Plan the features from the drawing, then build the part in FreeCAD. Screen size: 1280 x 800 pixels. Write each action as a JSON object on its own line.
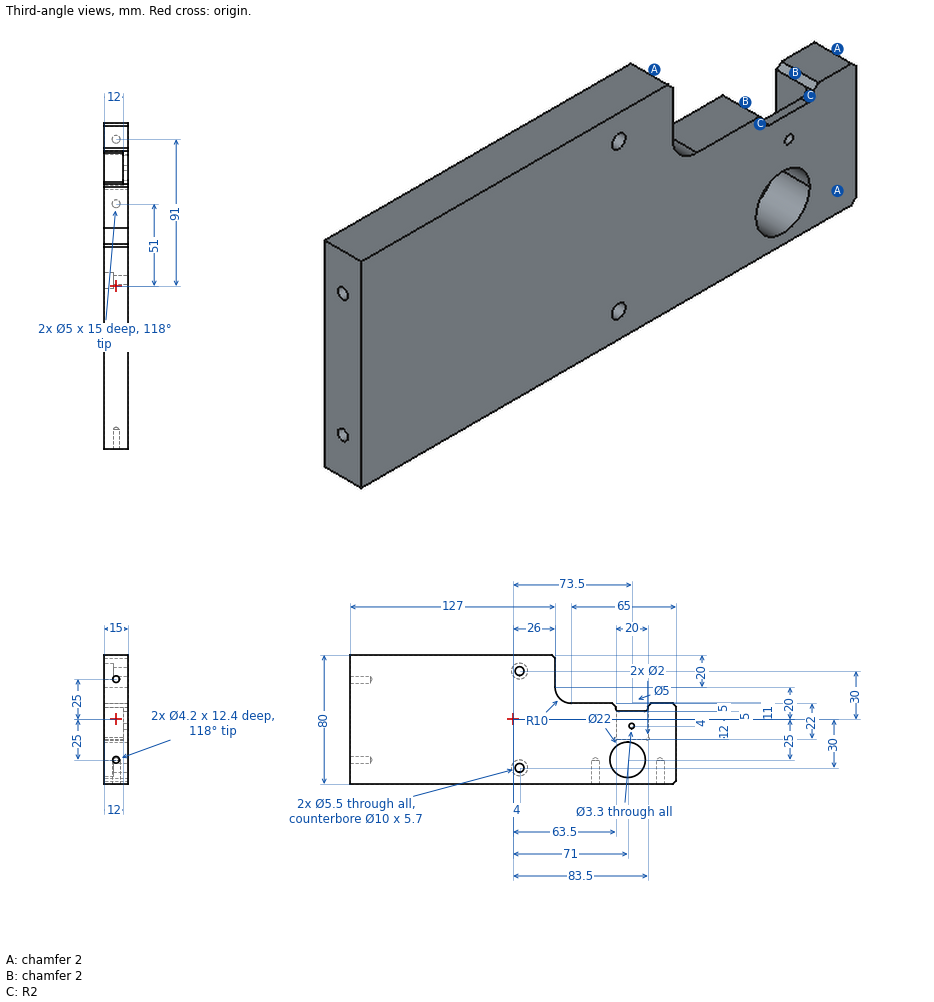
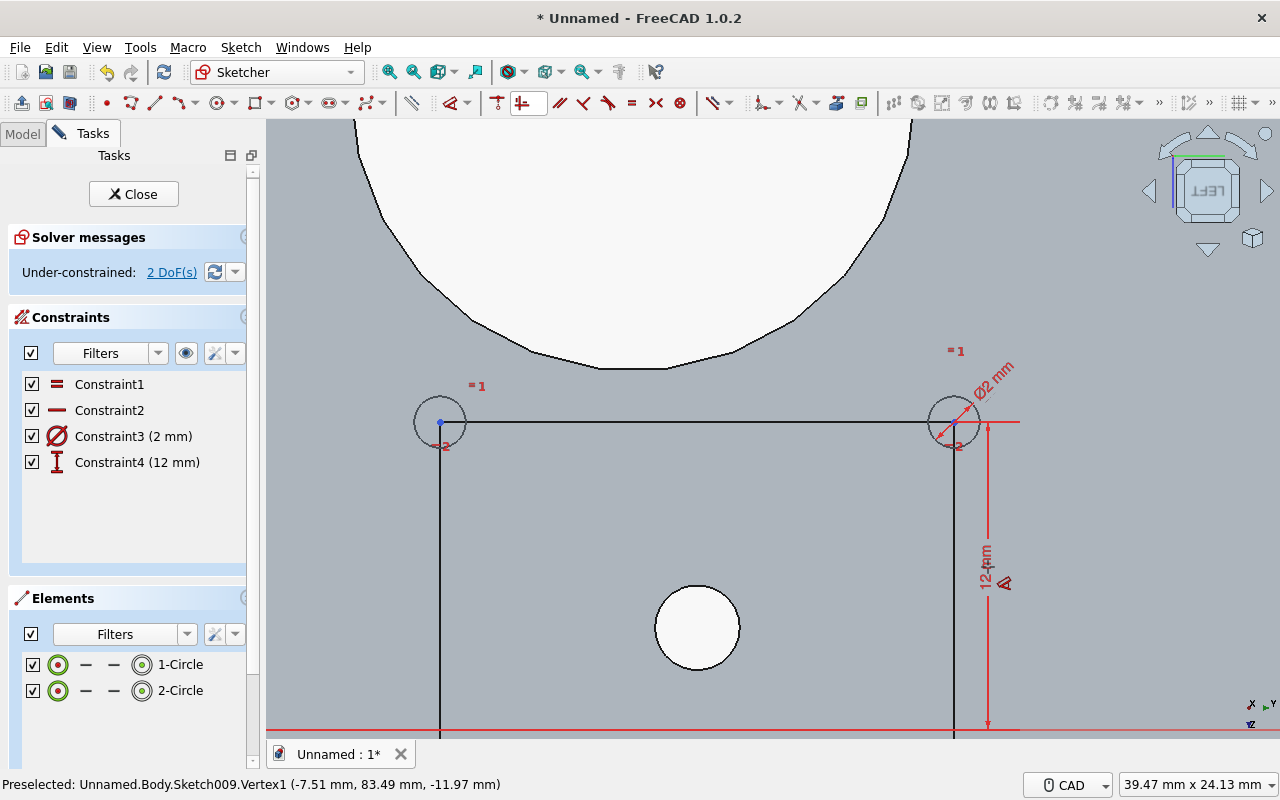
{"action": "left_click", "coordinate": [954, 422]}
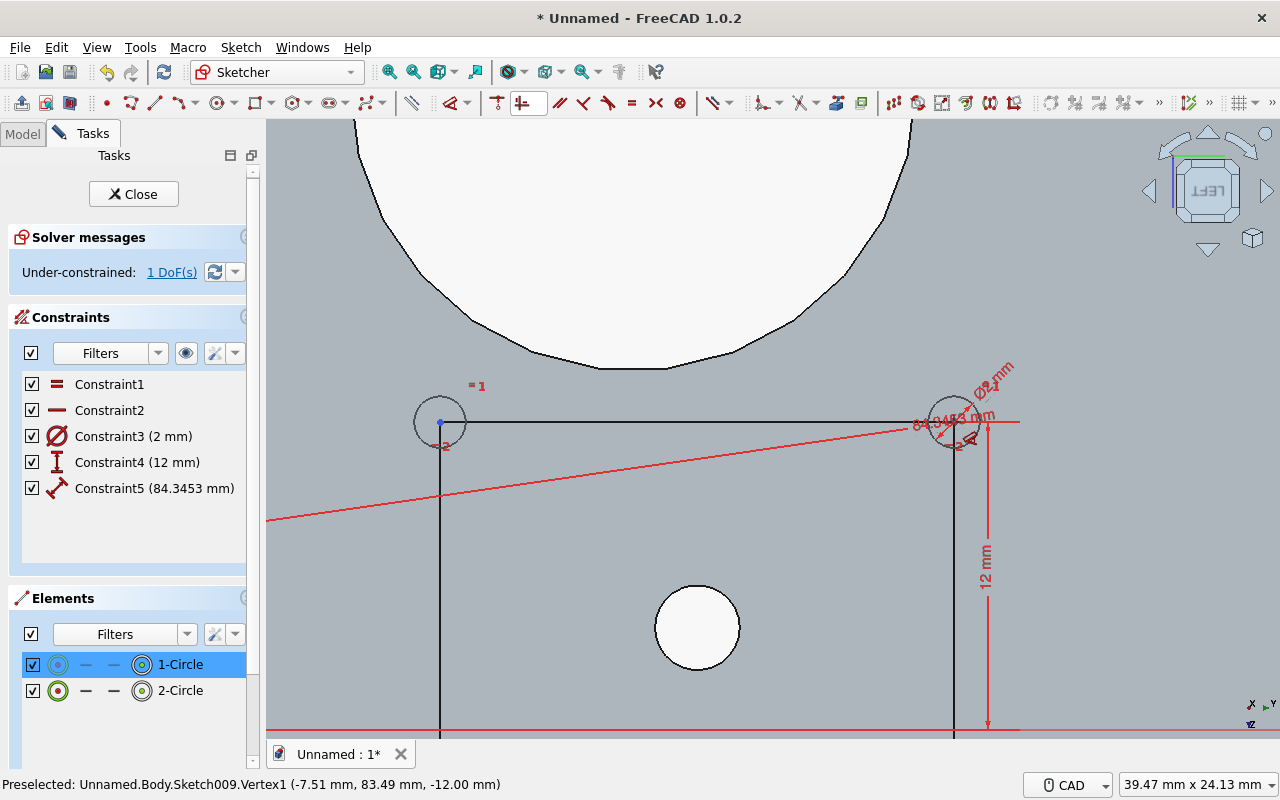
{"action": "left_click", "coordinate": [440, 422]}
{"action": "left_click", "coordinate": [697, 456]}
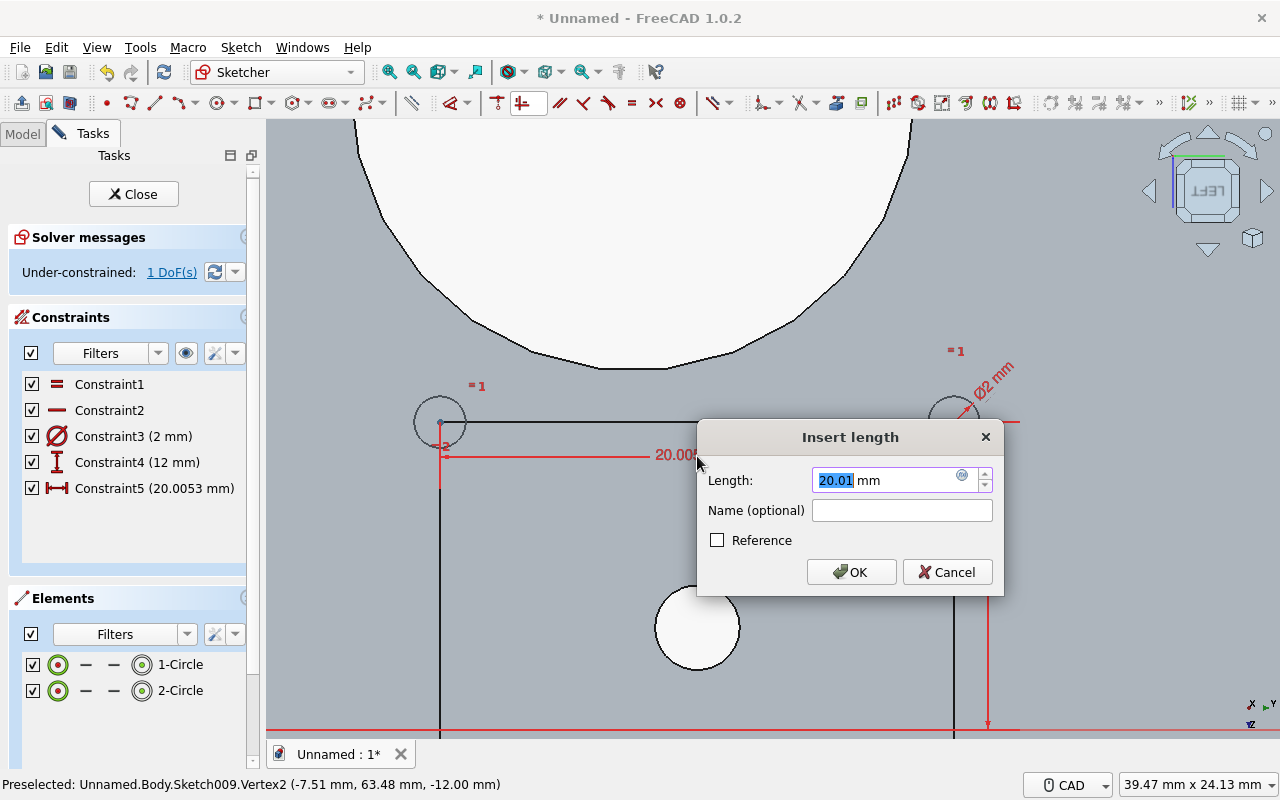
{"action": "type", "text": "20"}
{"action": "key", "text": "Return"}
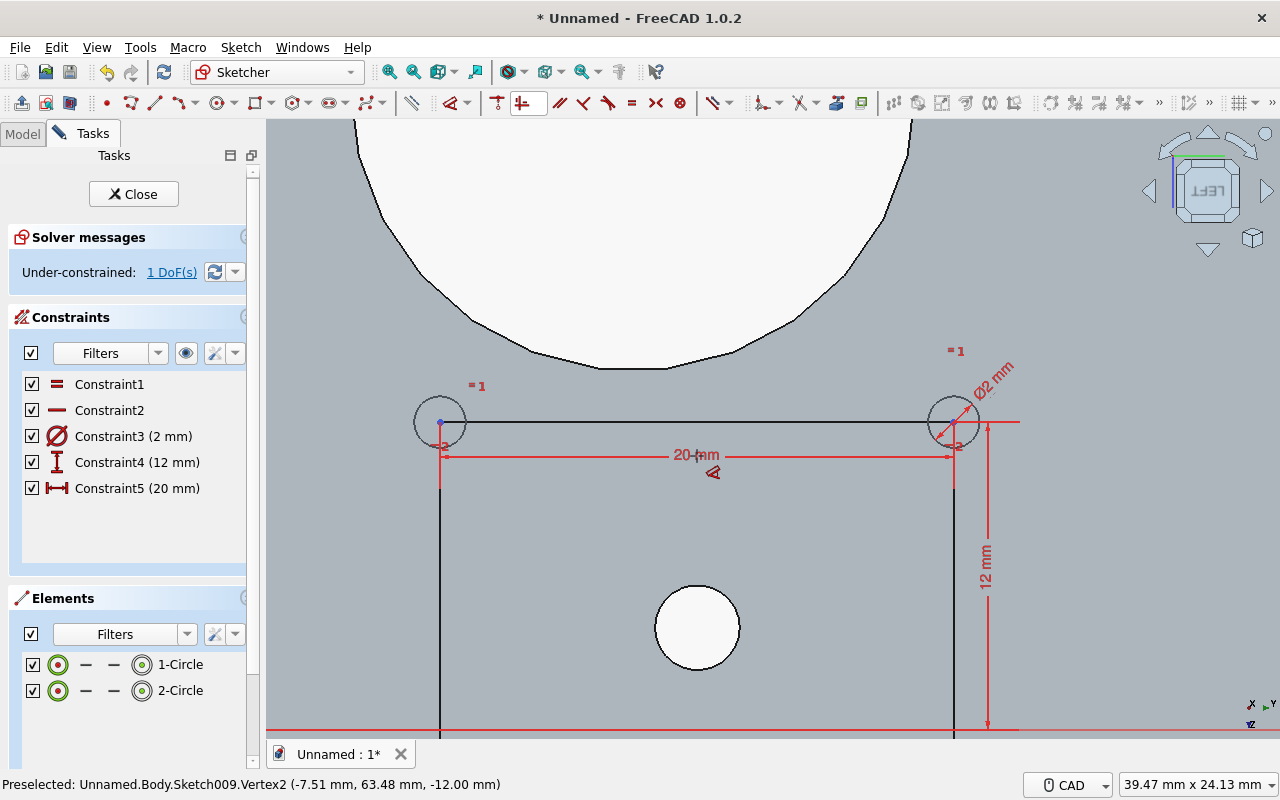
{"action": "left_click", "coordinate": [954, 422]}
{"action": "left_click", "coordinate": [624, 388]}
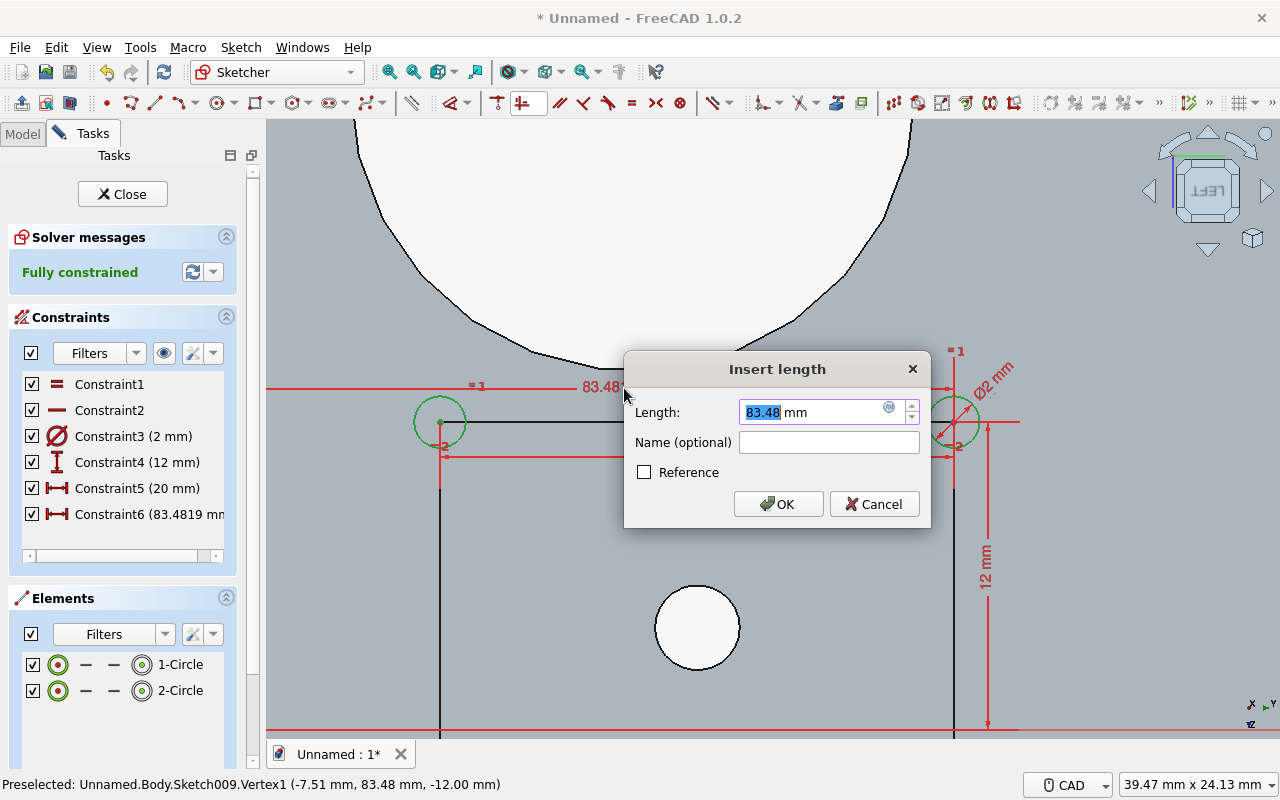
{"action": "type", "text": "83.5"}
{"action": "key", "text": "Return"}
{"action": "key", "text": "Escape"}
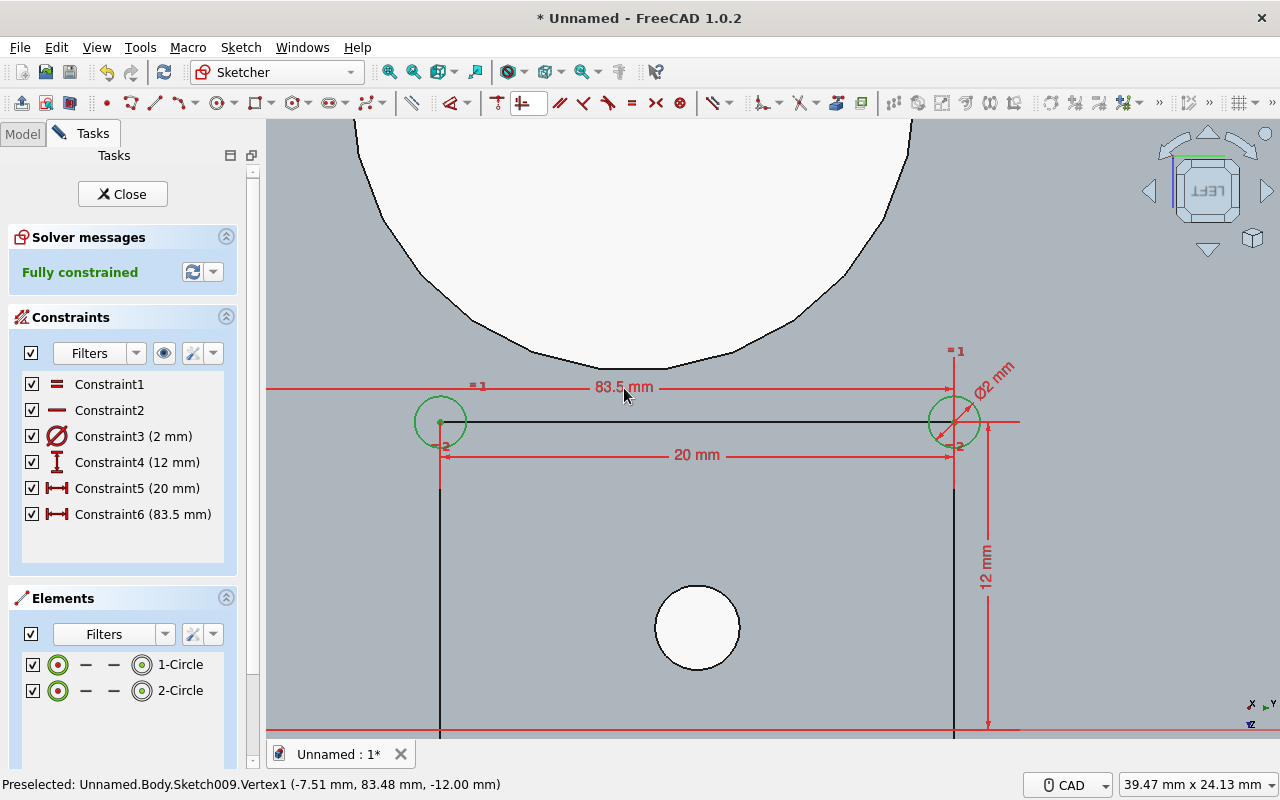
{"action": "left_click", "coordinate": [123, 194]}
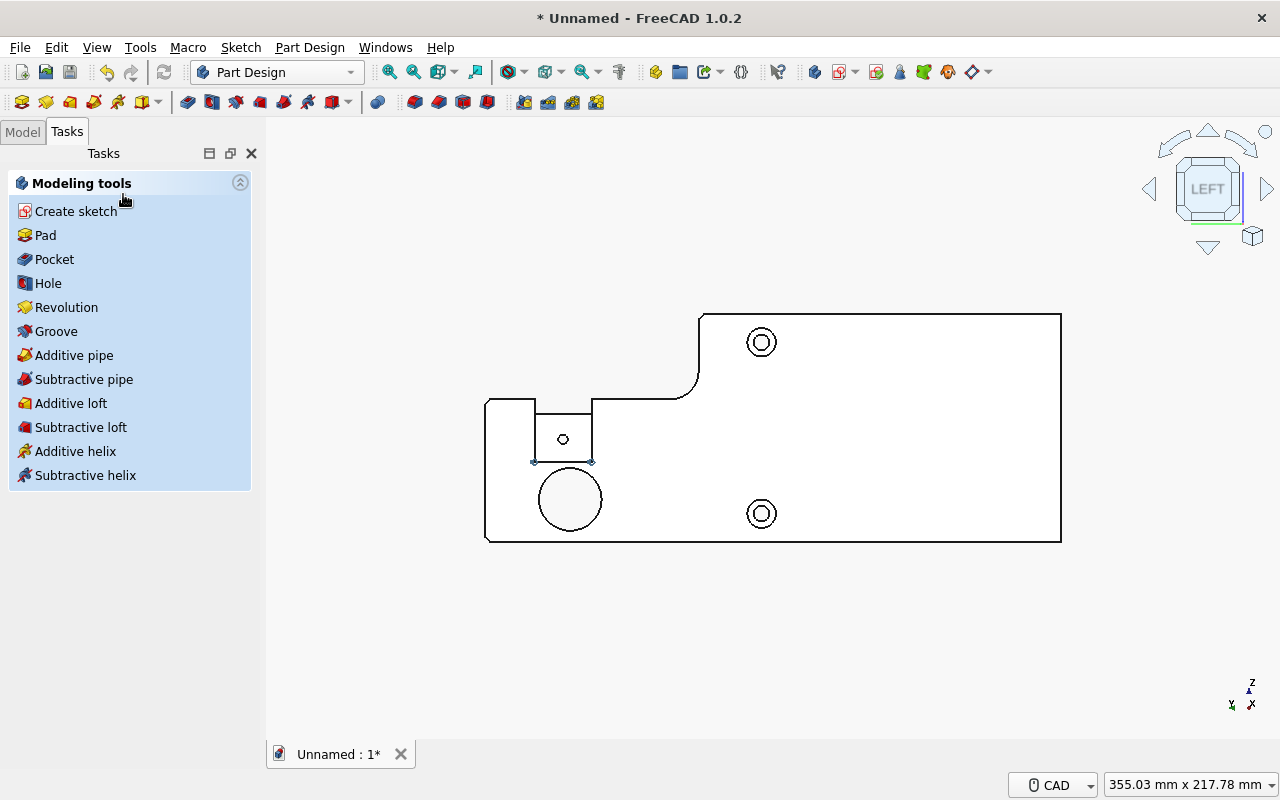
{"action": "left_click", "coordinate": [188, 102]}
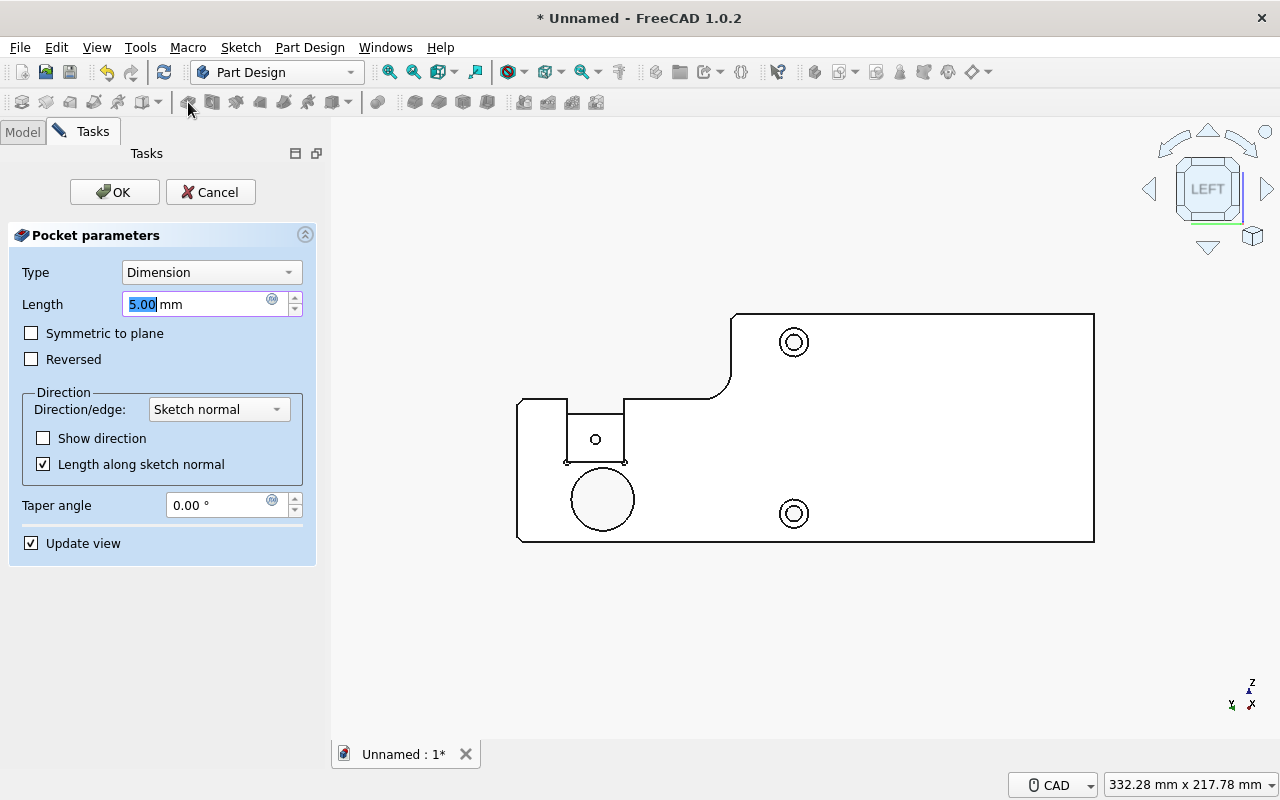
{"action": "type", "text": "12"}
{"action": "key", "text": "Tab"}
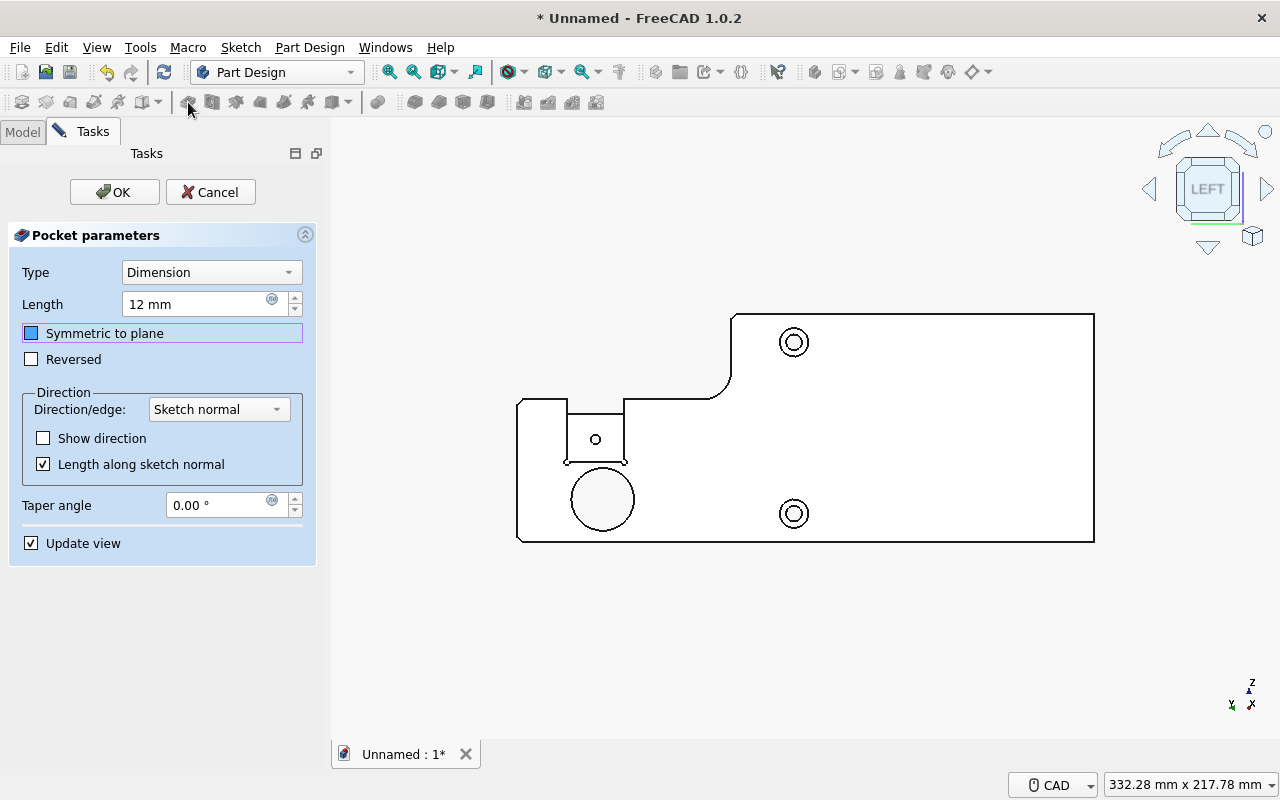
{"action": "left_click", "coordinate": [115, 192]}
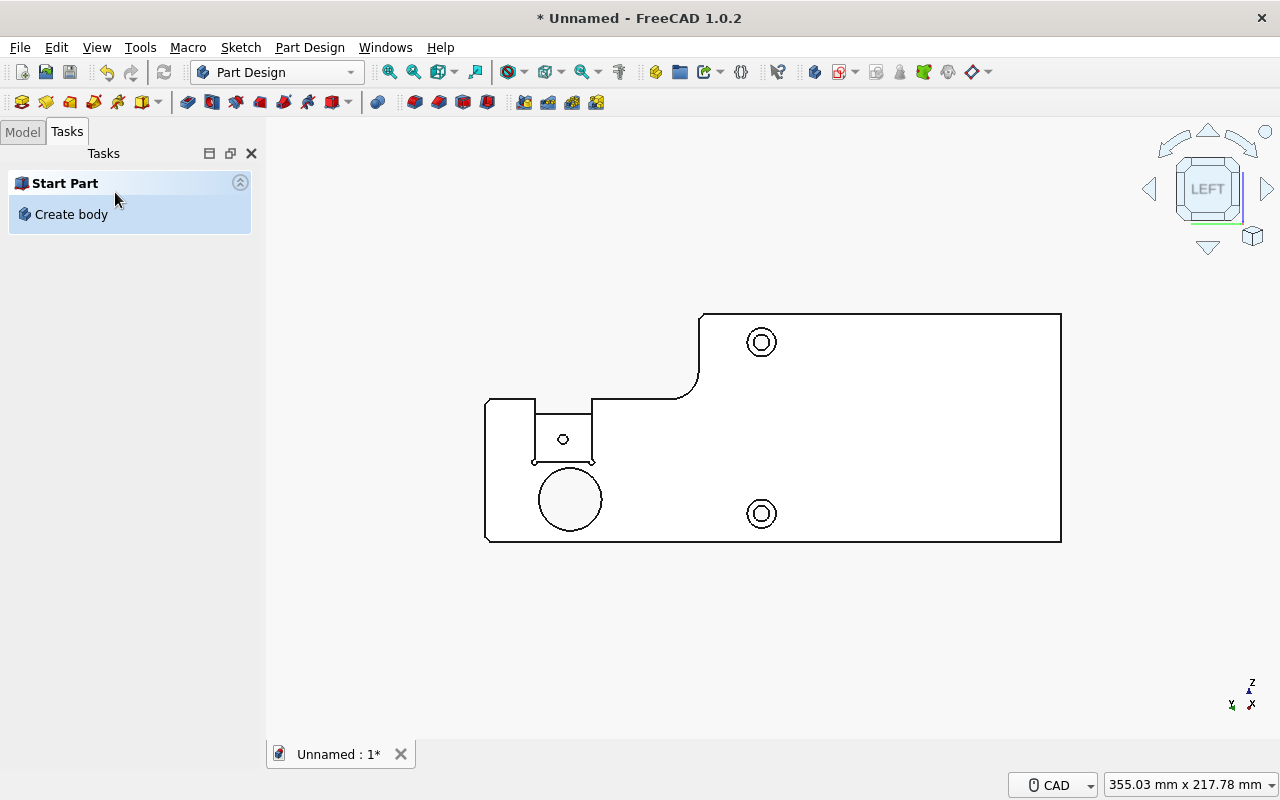
{"action": "key", "text": "0"}